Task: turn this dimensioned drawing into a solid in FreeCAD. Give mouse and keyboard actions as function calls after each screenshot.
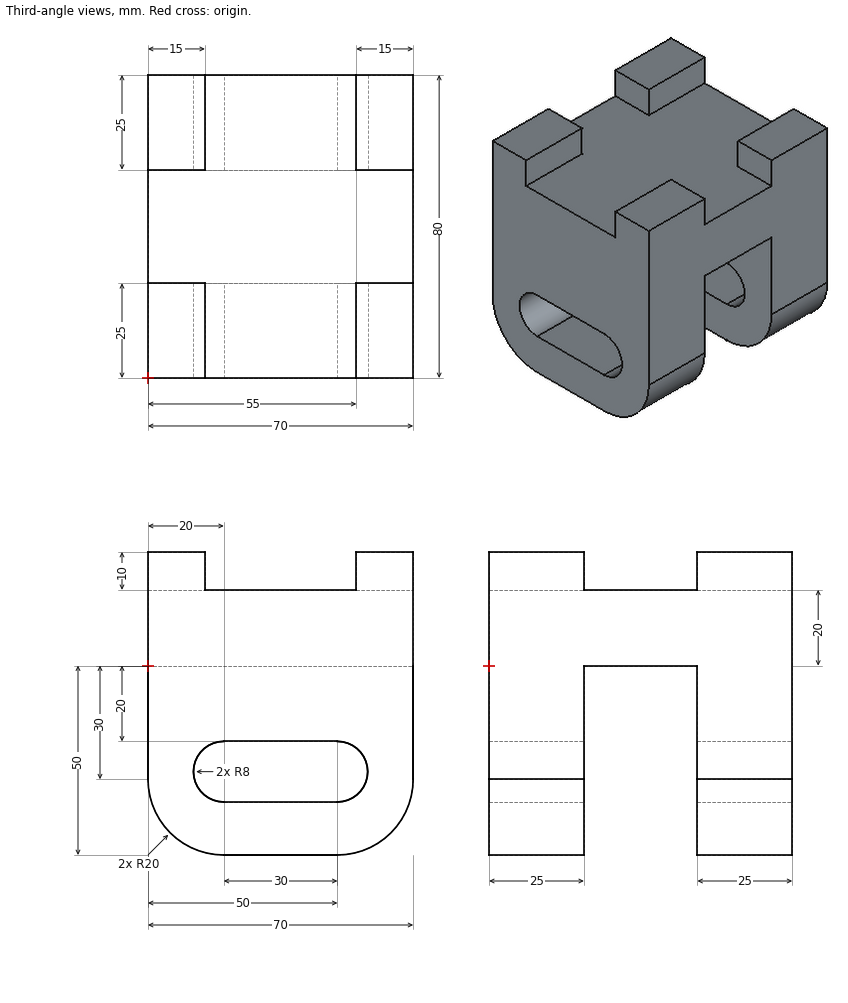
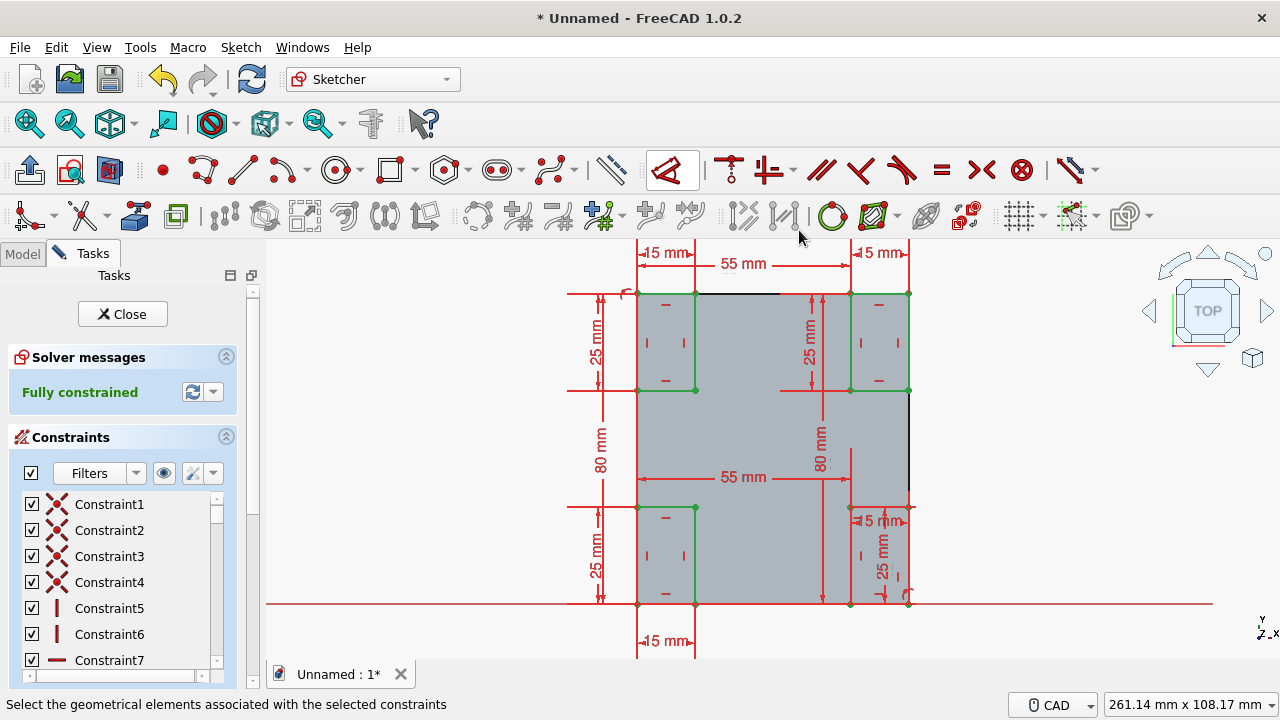
click(123, 314)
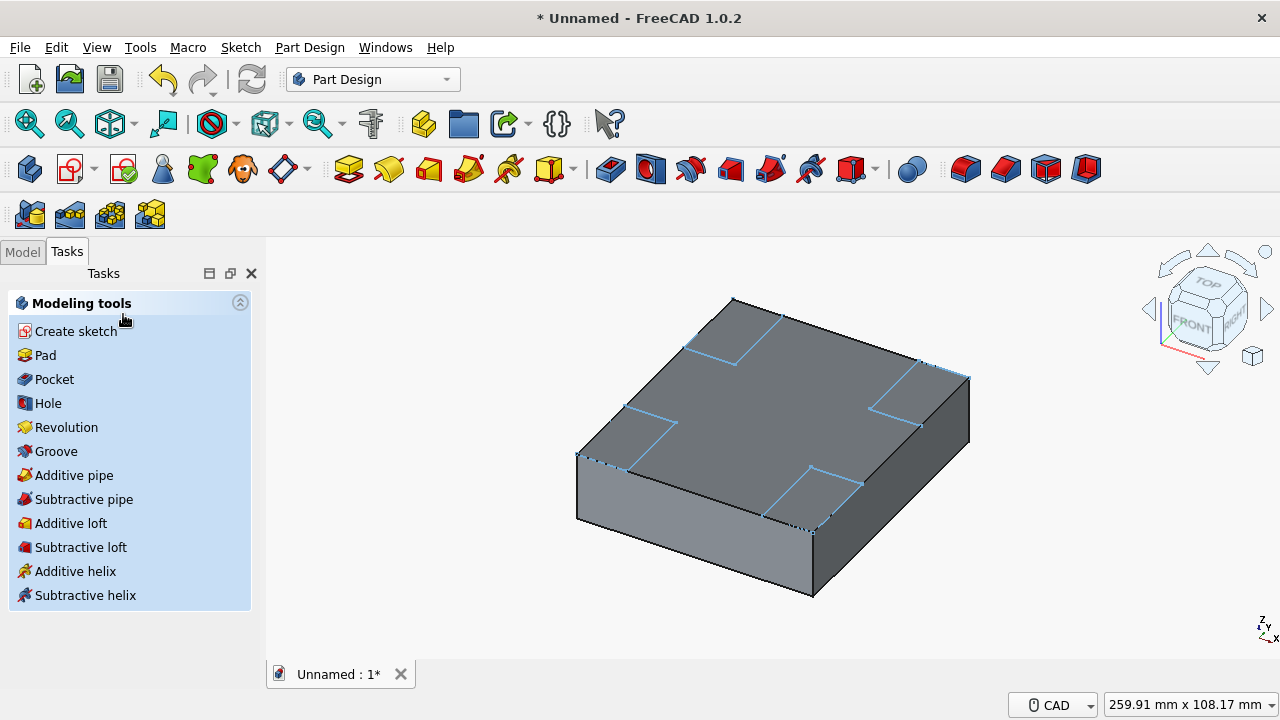
click(350, 170)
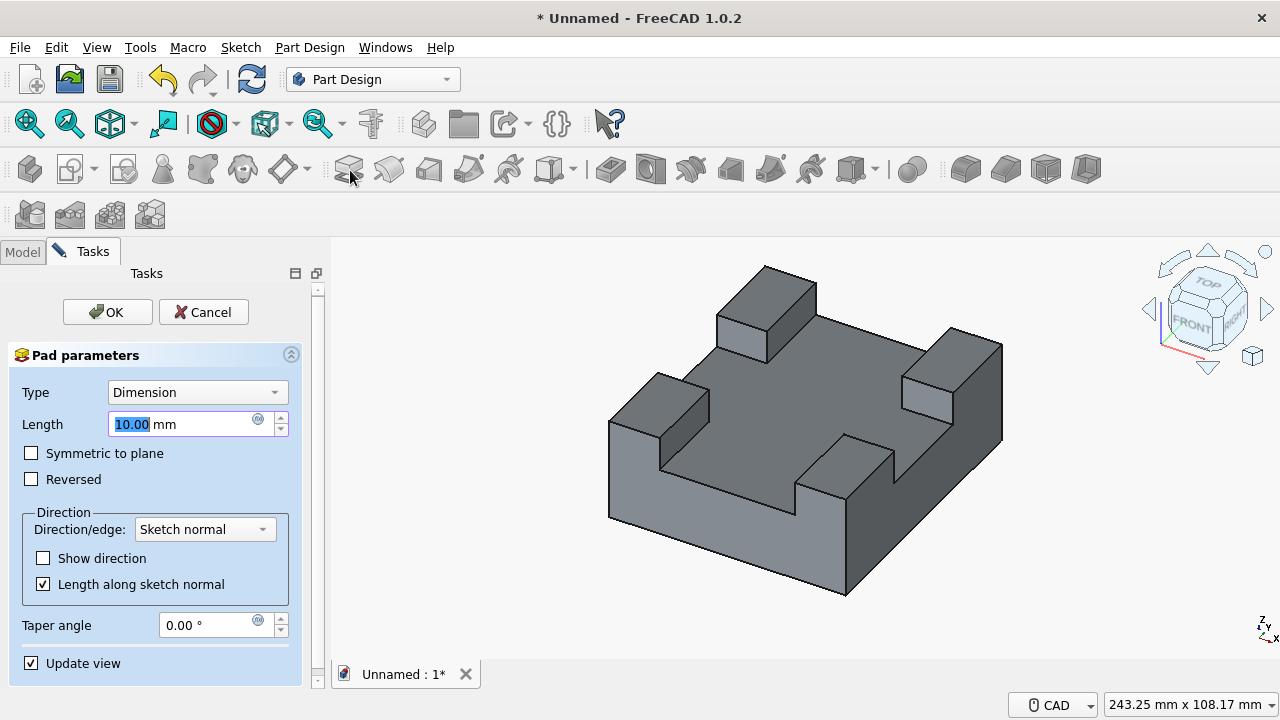
text(10)
key(Tab)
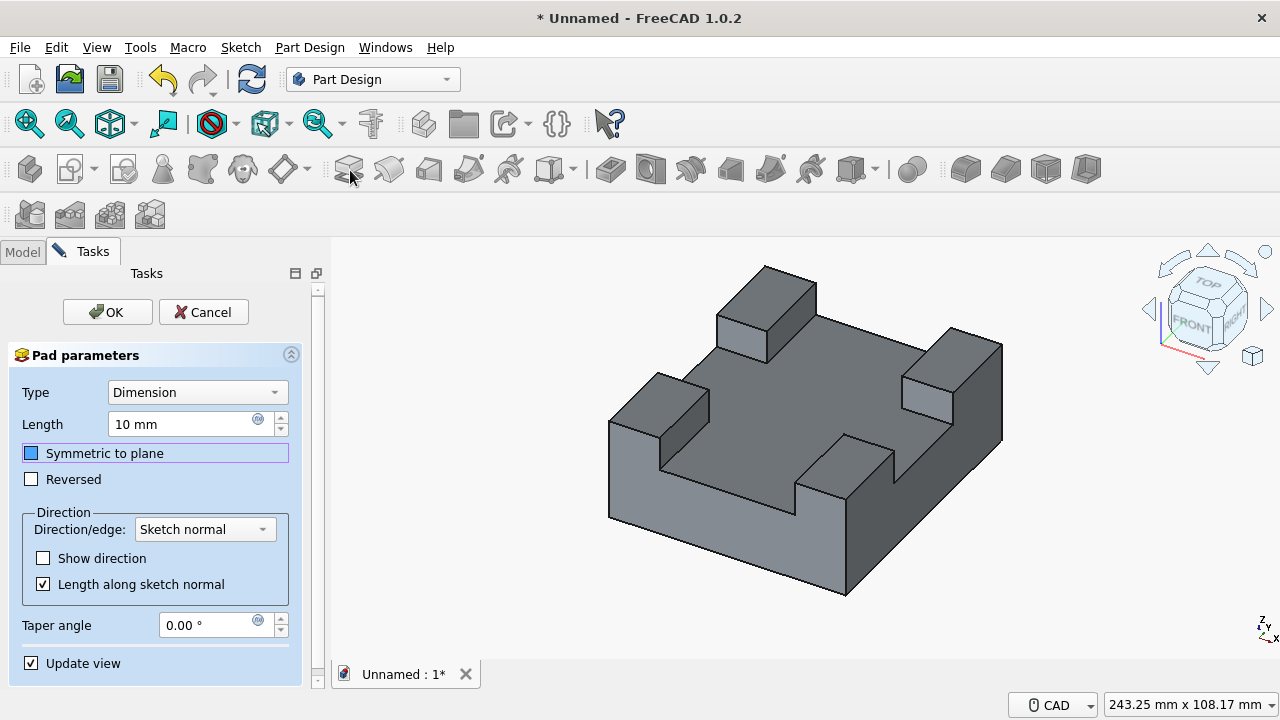
click(108, 312)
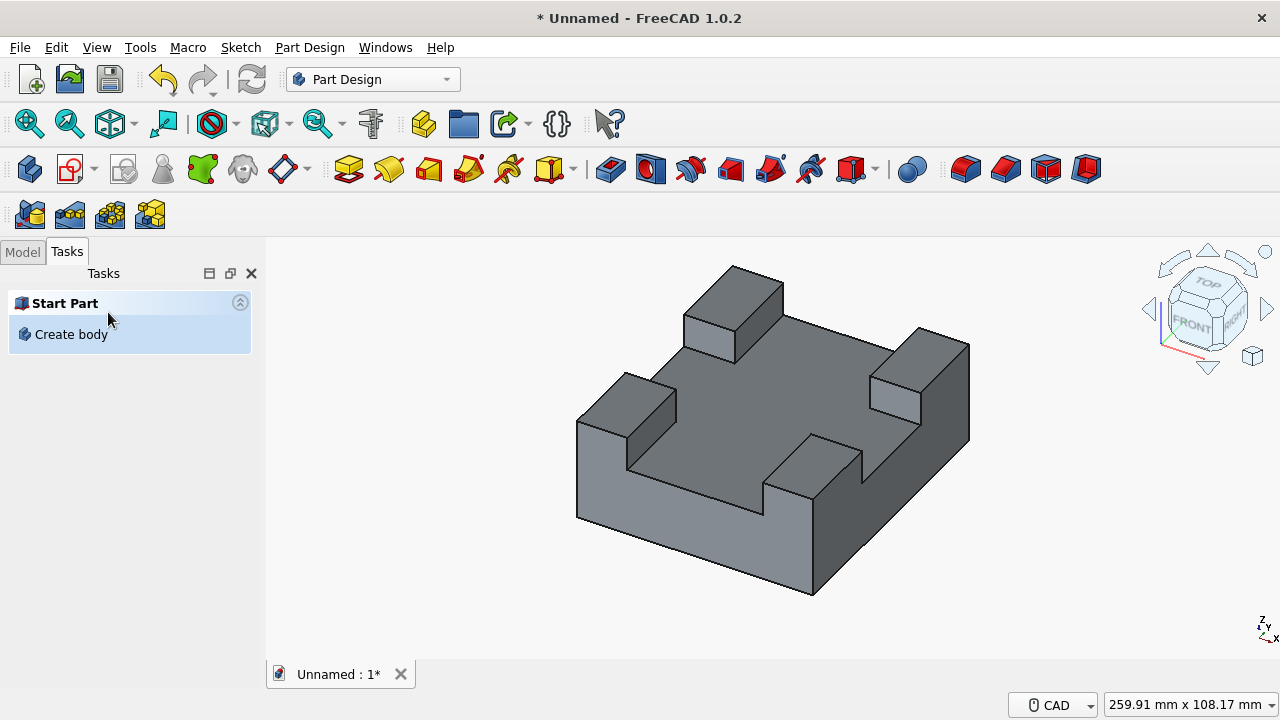
key(4)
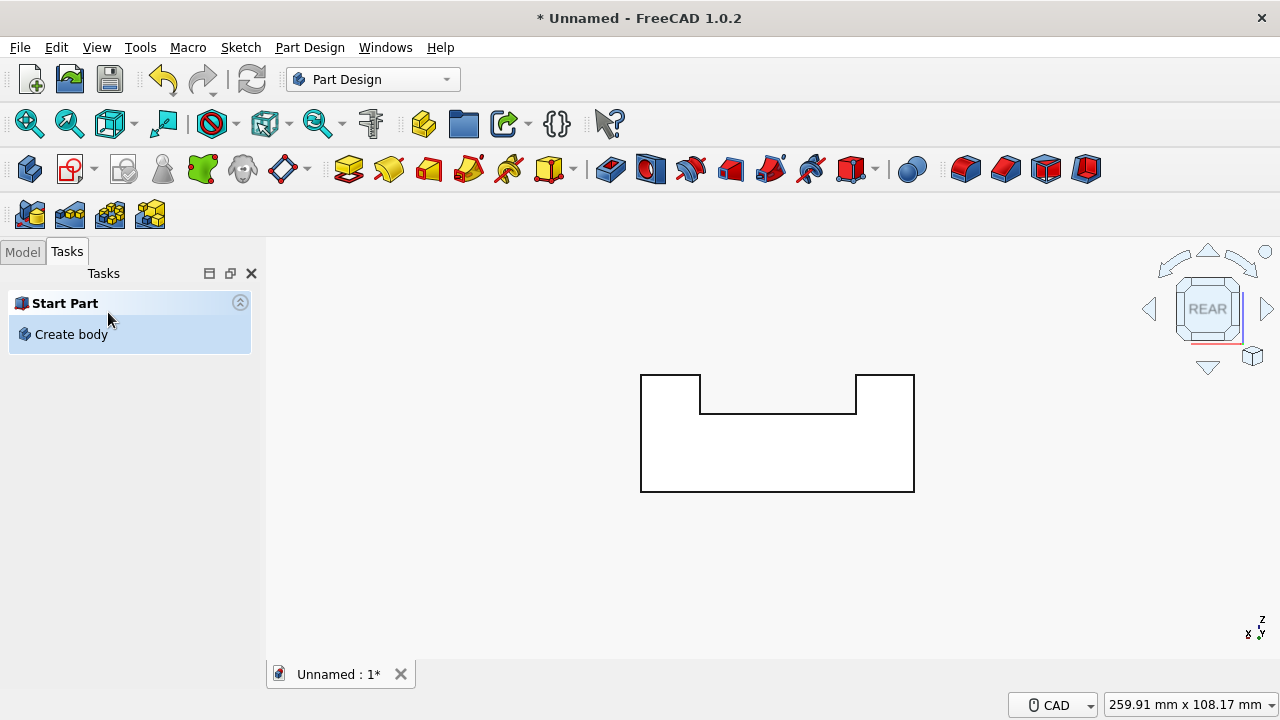
click(30, 124)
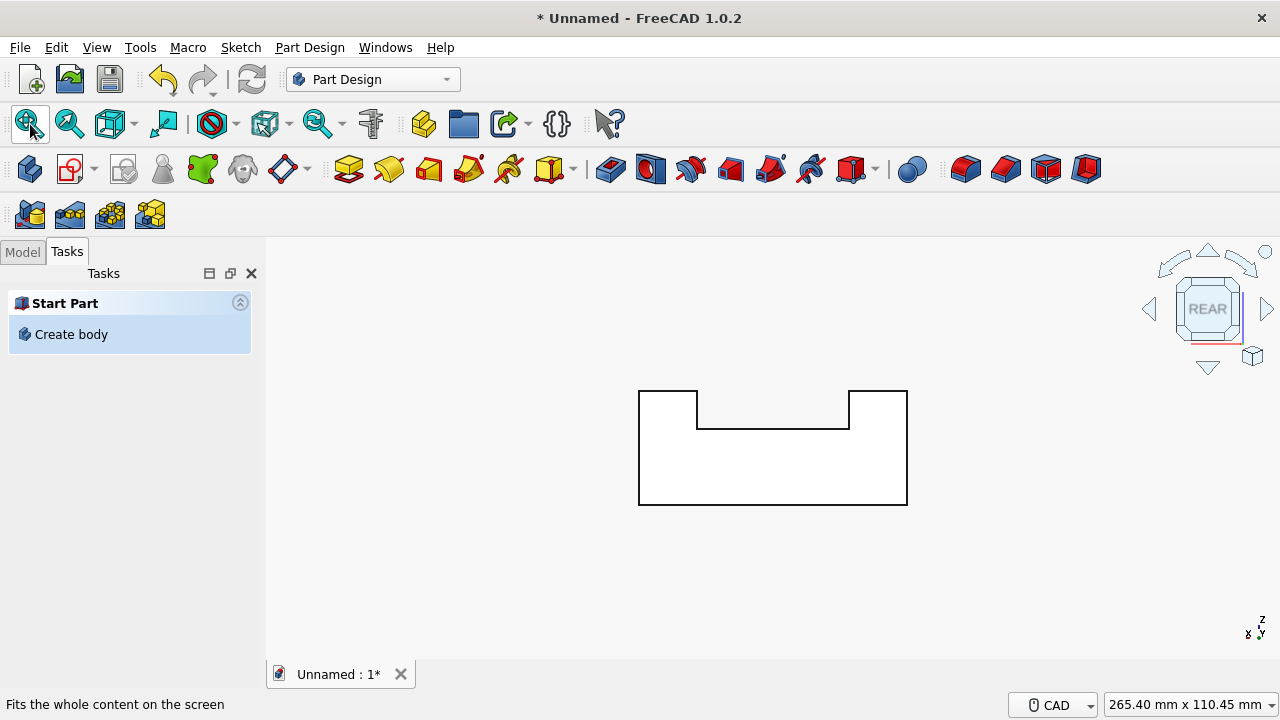
click(697, 463)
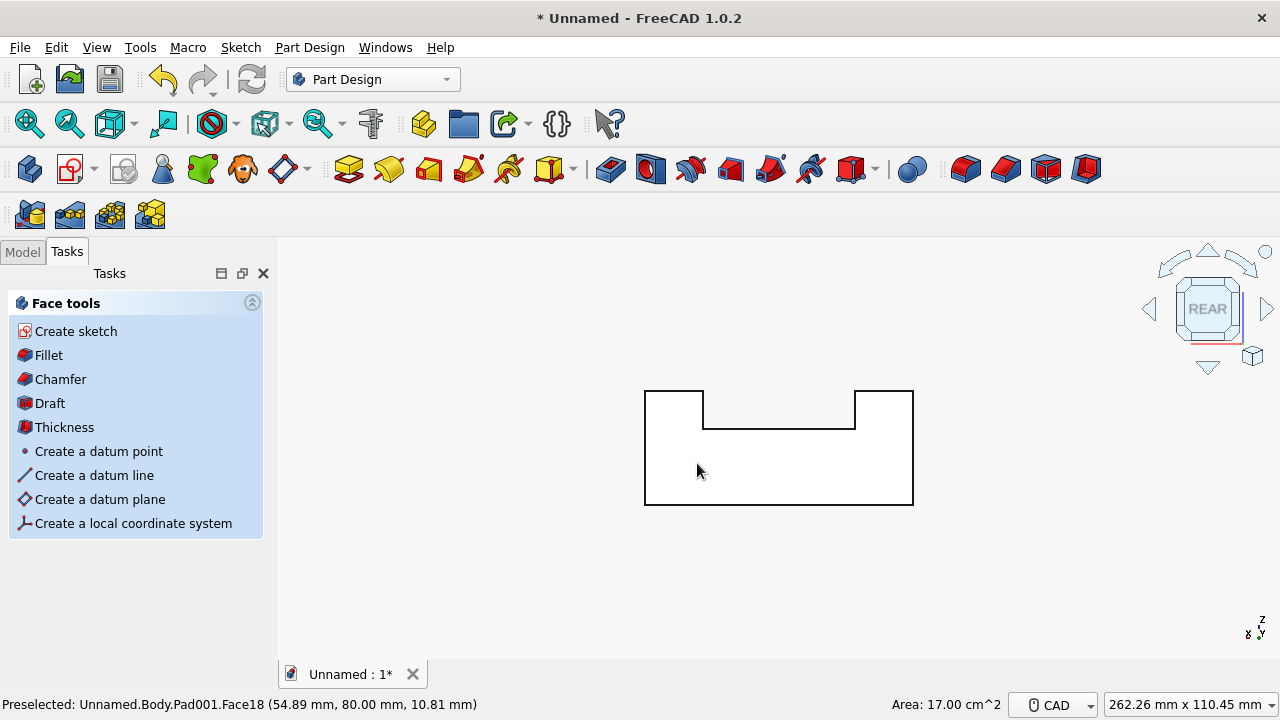
click(70, 170)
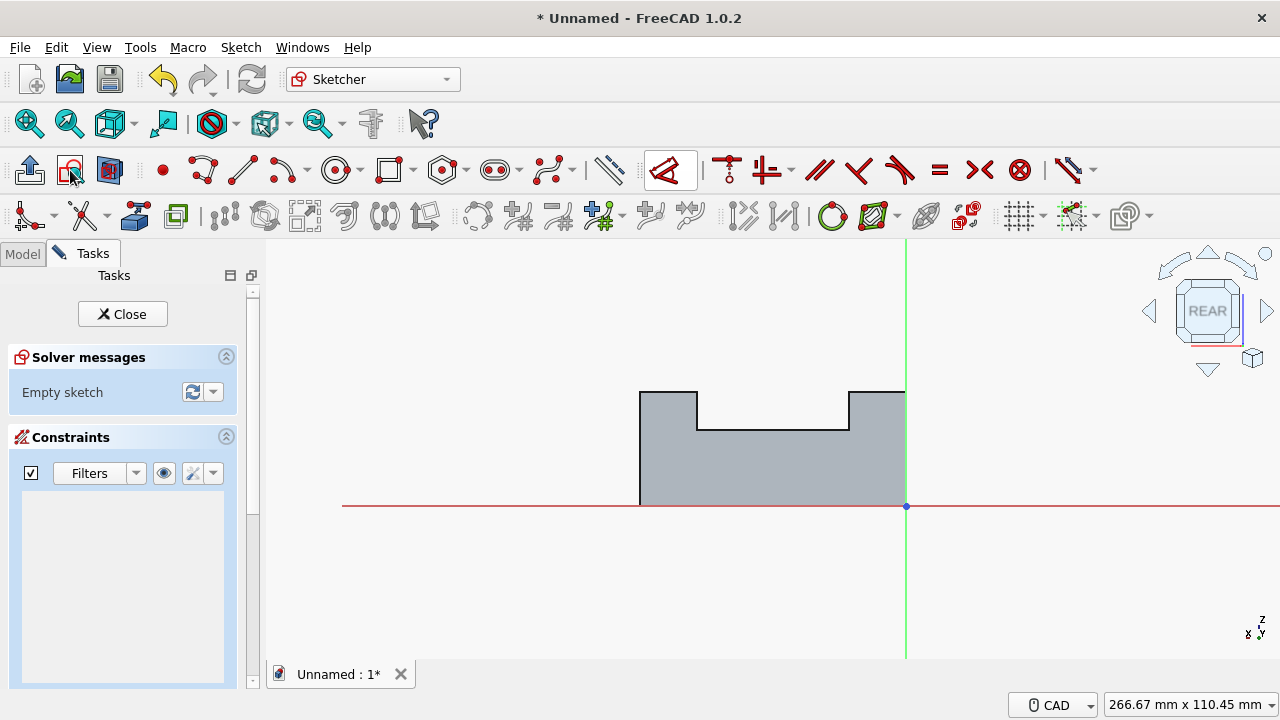
scroll(704, 449, down, 5)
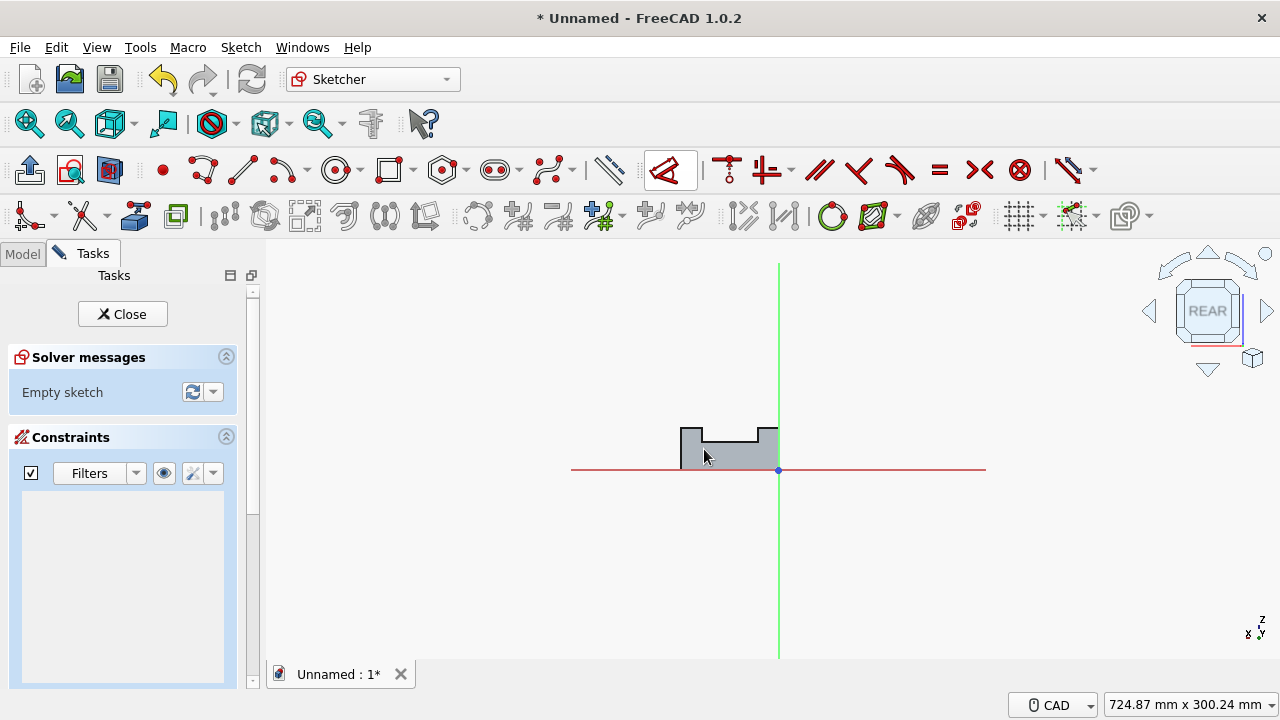
scroll(738, 524, up, 7)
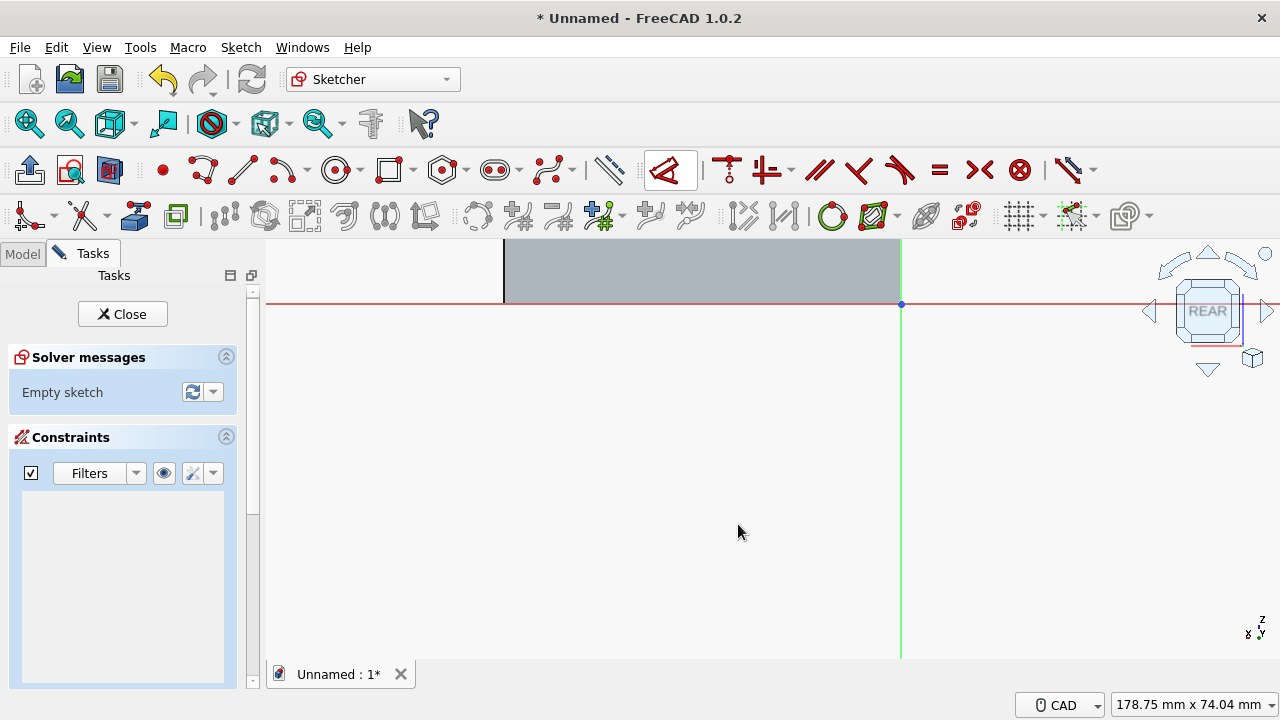
click(390, 170)